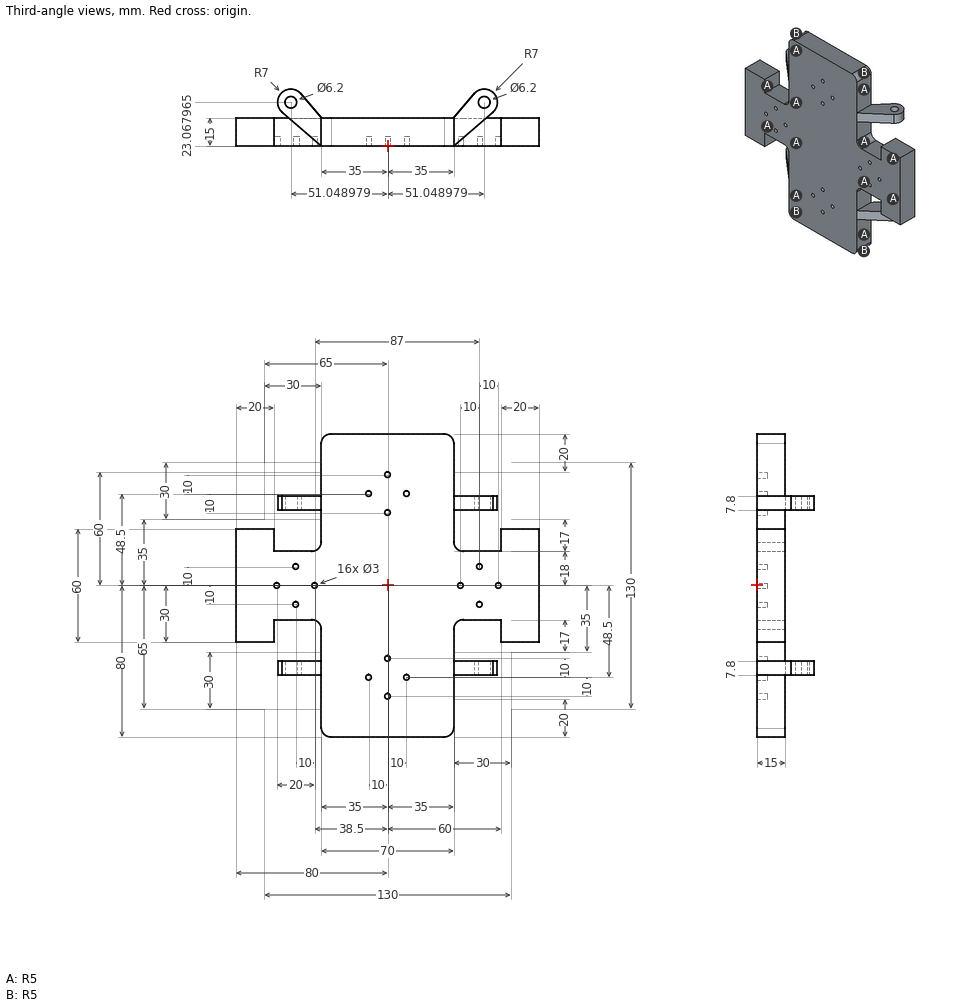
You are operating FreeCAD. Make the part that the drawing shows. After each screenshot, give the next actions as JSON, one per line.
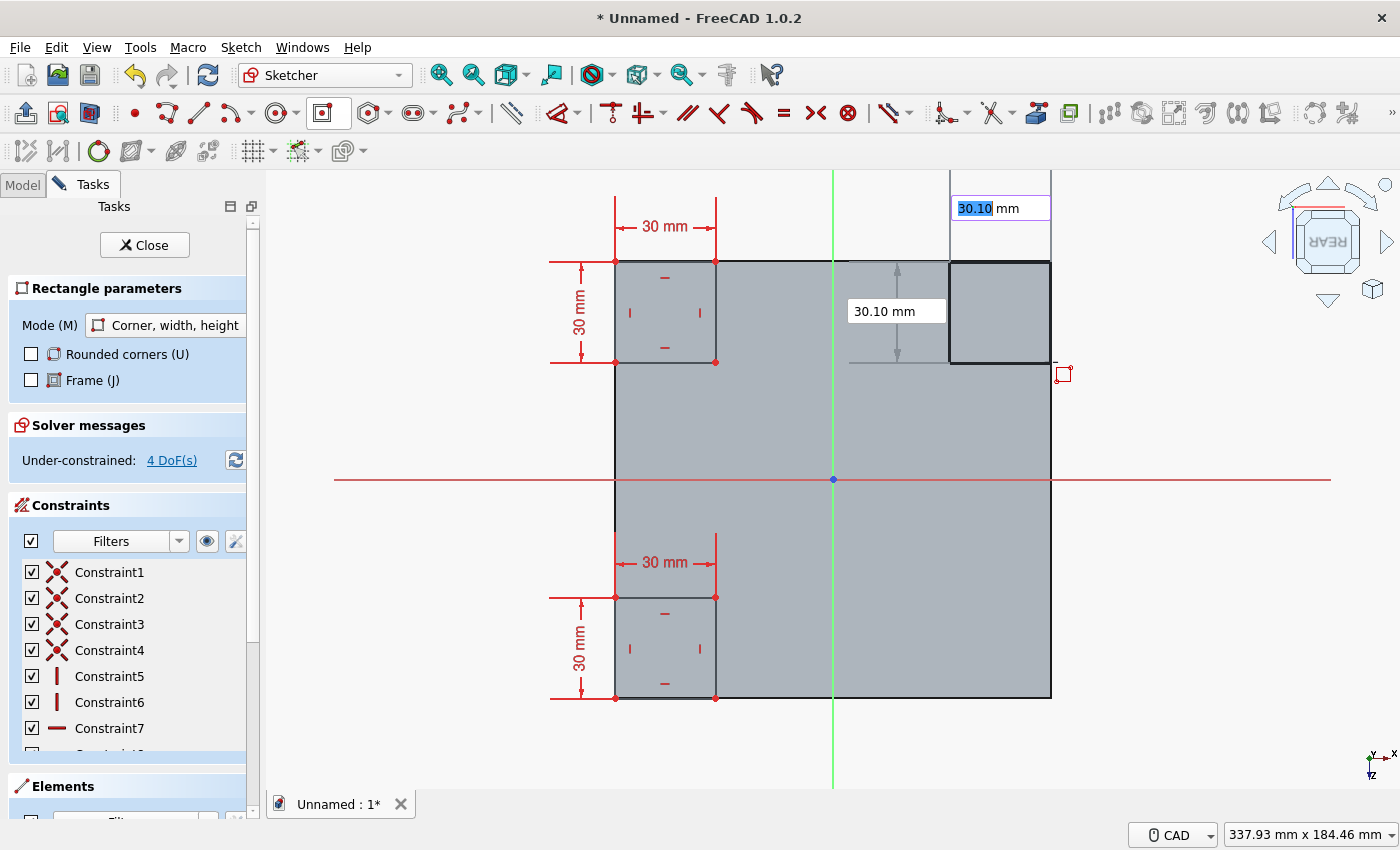
{"action": "type", "text": "30"}
{"action": "key", "text": "Tab"}
{"action": "type", "text": "30"}
{"action": "key", "text": "Return"}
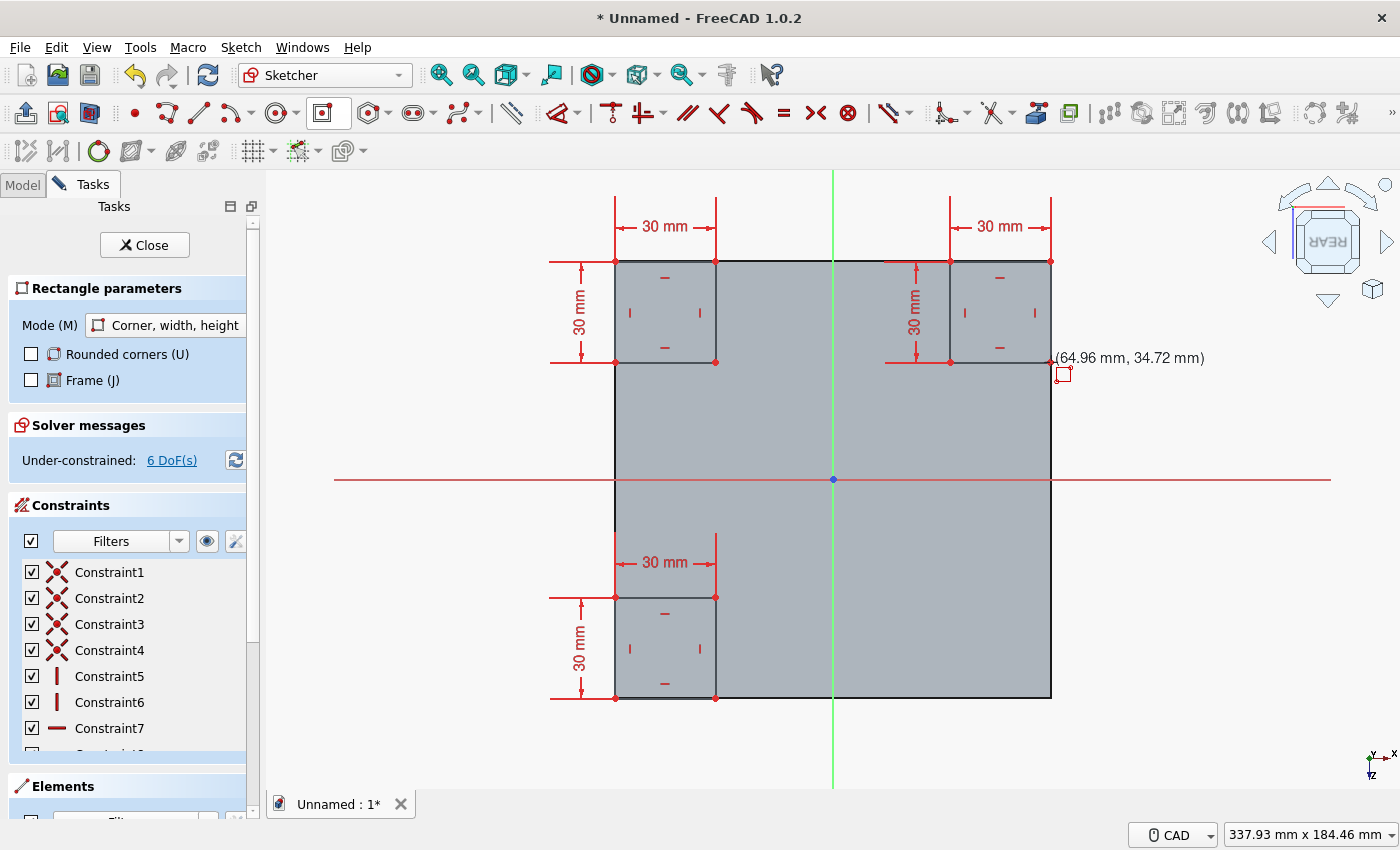
{"action": "left_click", "coordinate": [950, 597]}
{"action": "mouse_move", "coordinate": [1051, 698]}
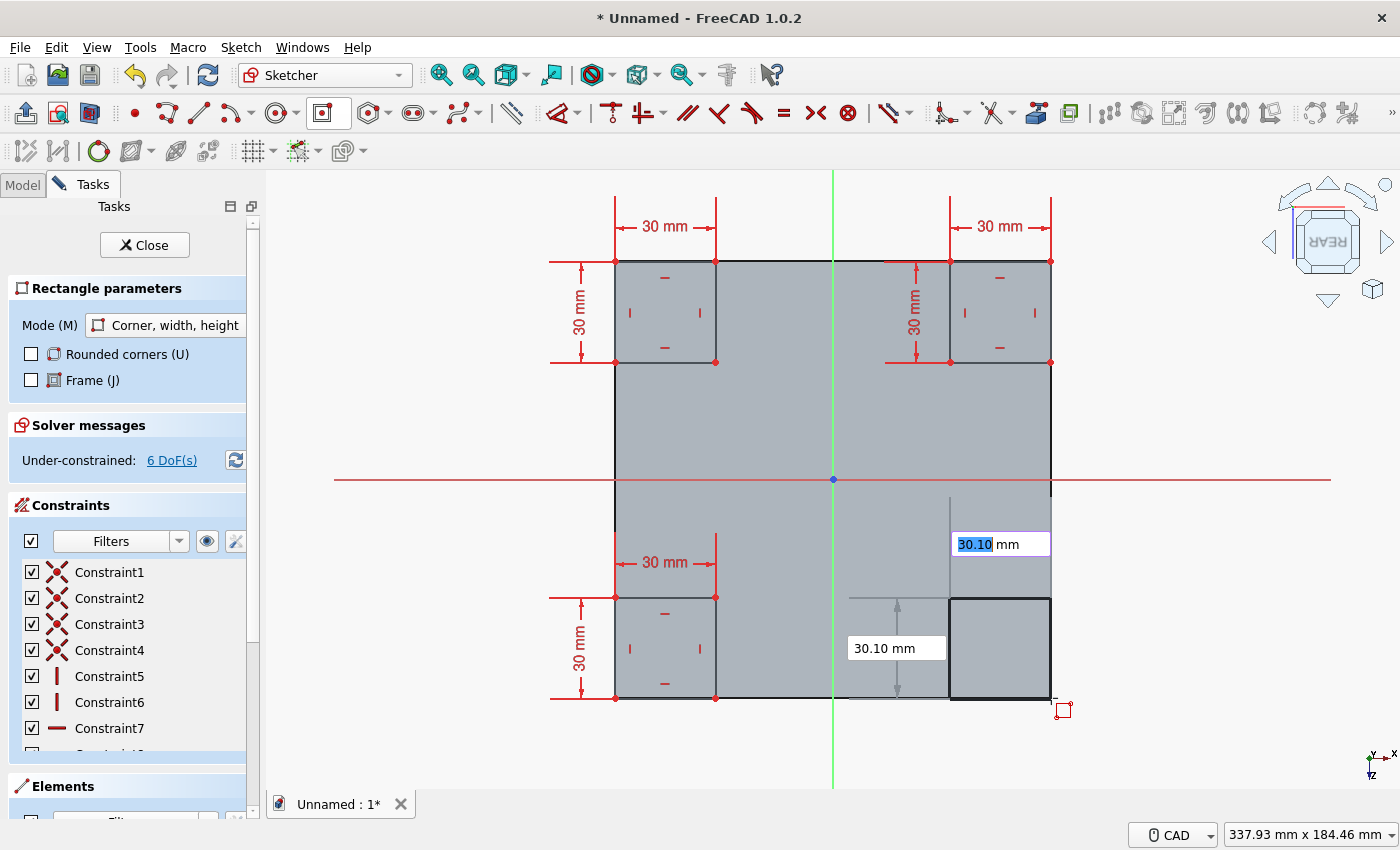
{"action": "type", "text": "30"}
{"action": "key", "text": "Tab"}
{"action": "type", "text": "30"}
{"action": "key", "text": "Return"}
{"action": "key", "text": "Escape"}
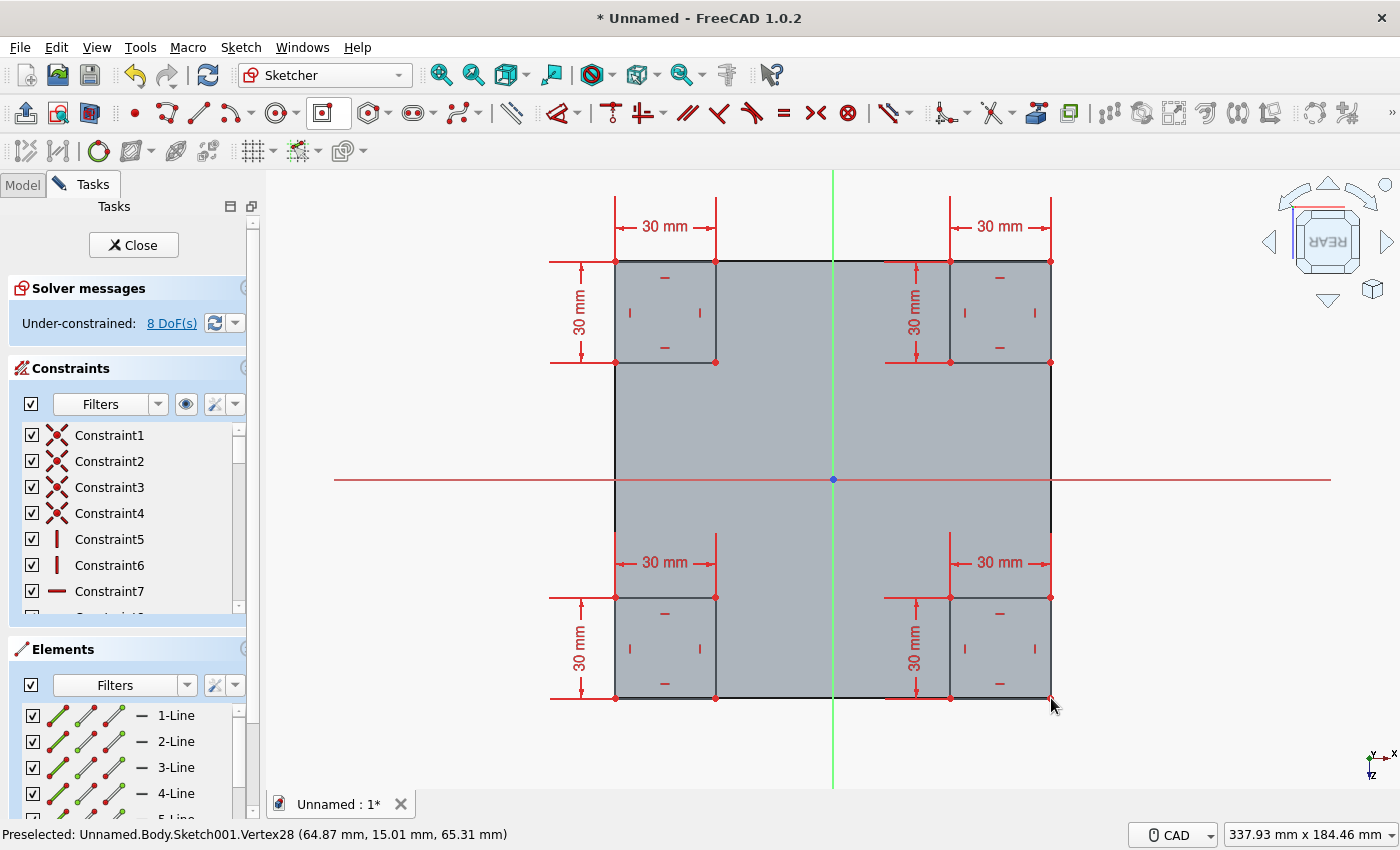
{"action": "key", "text": "d"}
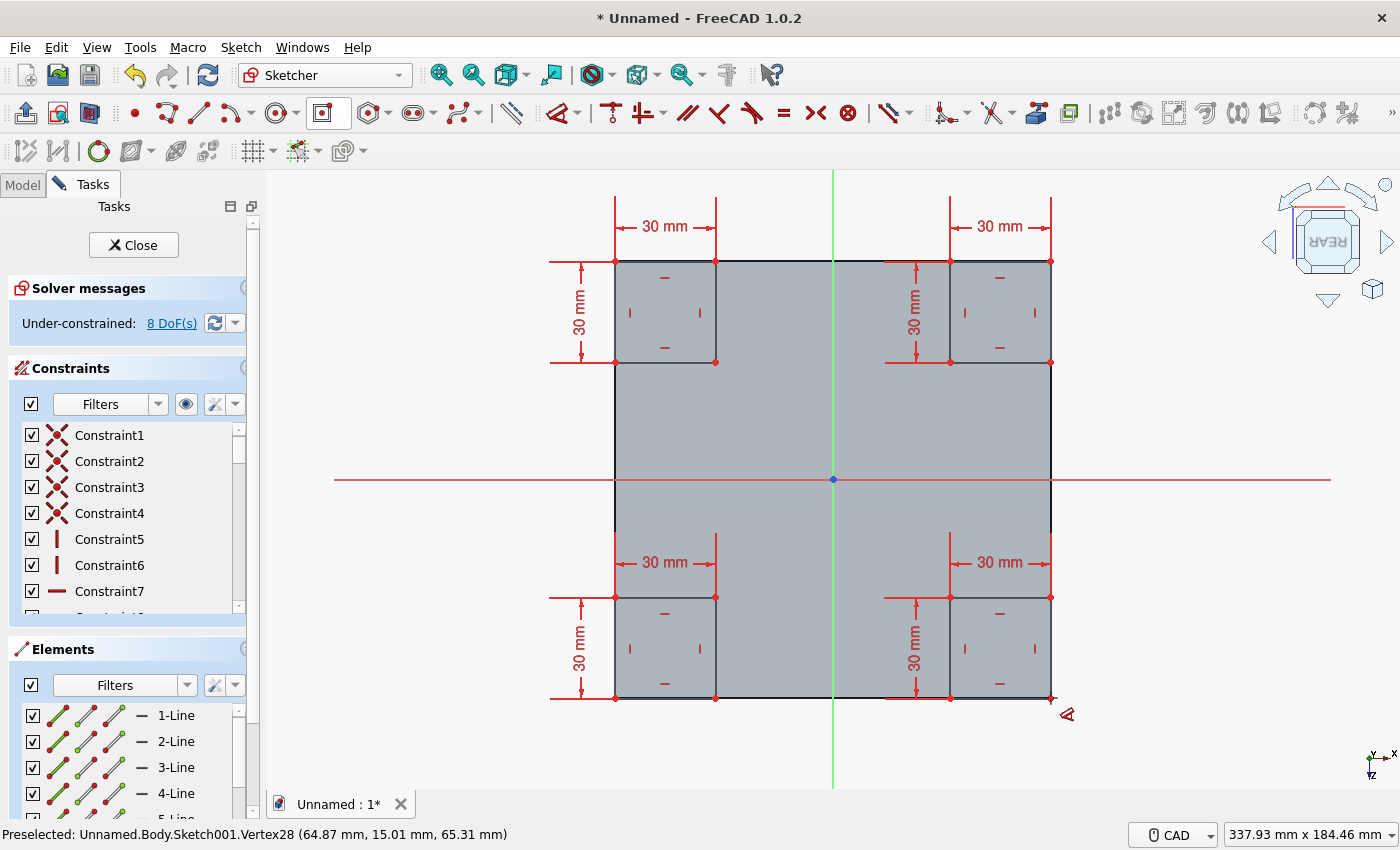
{"action": "left_click", "coordinate": [615, 598]}
{"action": "left_click", "coordinate": [674, 632]}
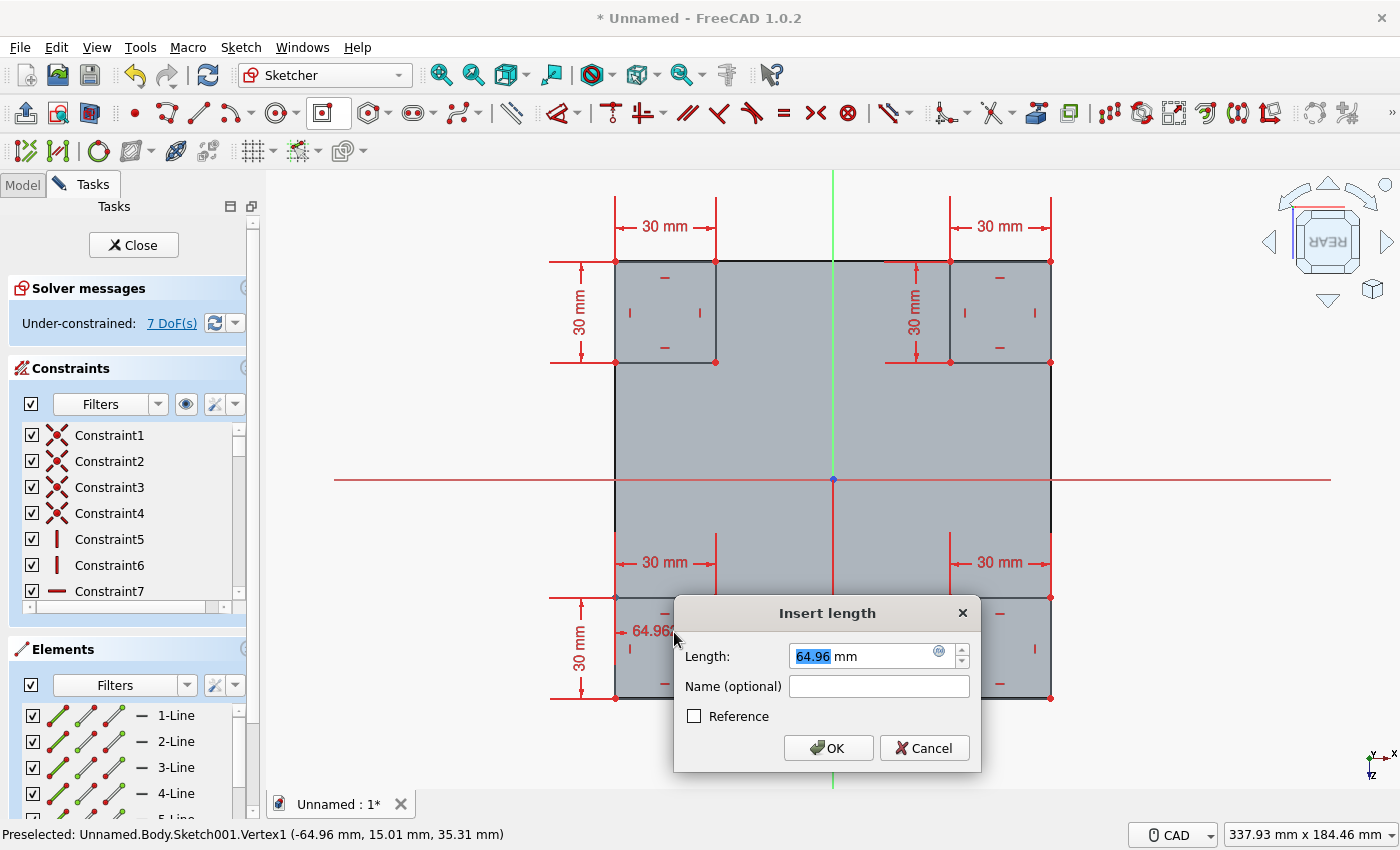
{"action": "type", "text": "65"}
{"action": "key", "text": "Return"}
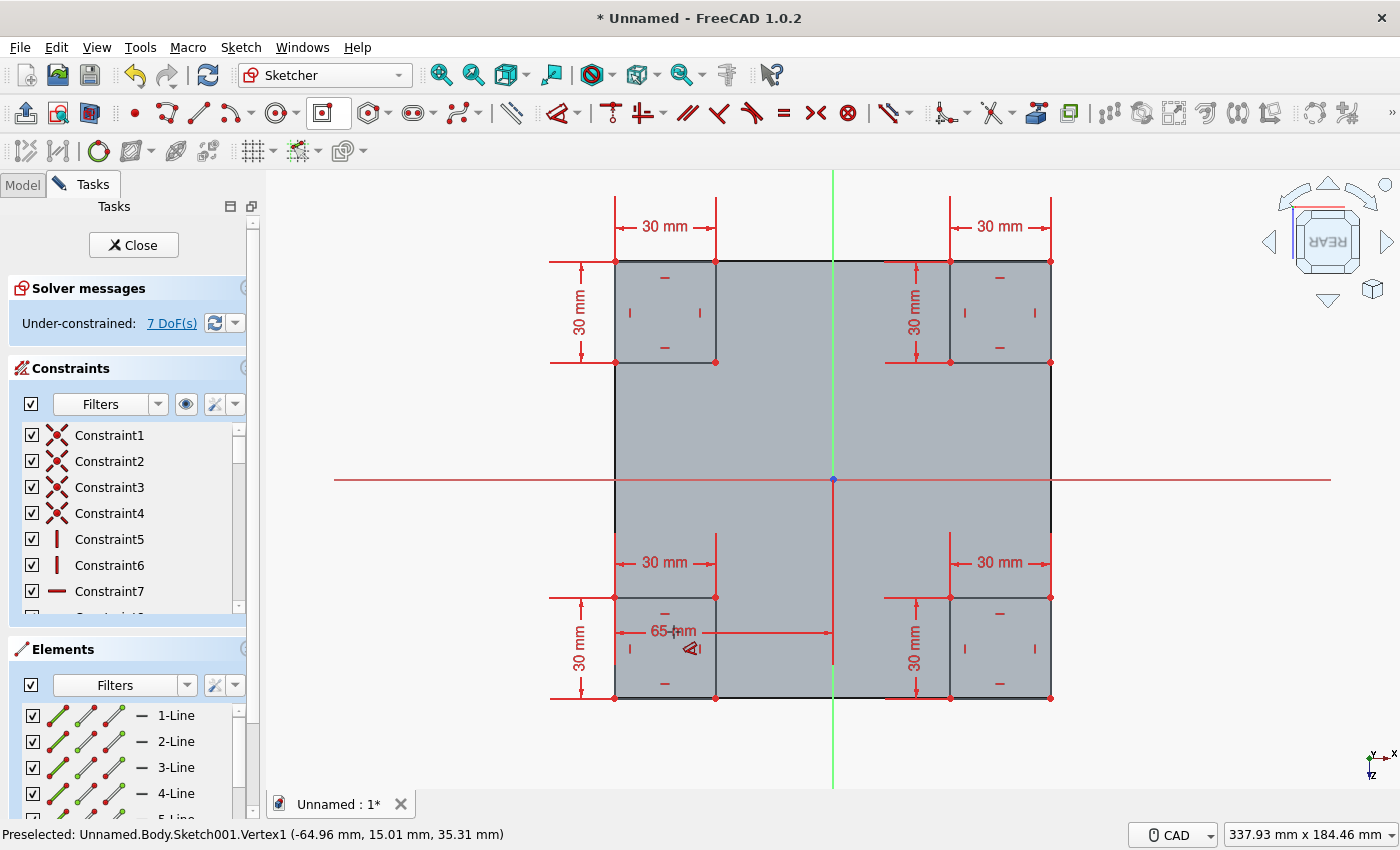
{"action": "left_click", "coordinate": [615, 598]}
{"action": "left_click", "coordinate": [581, 539]}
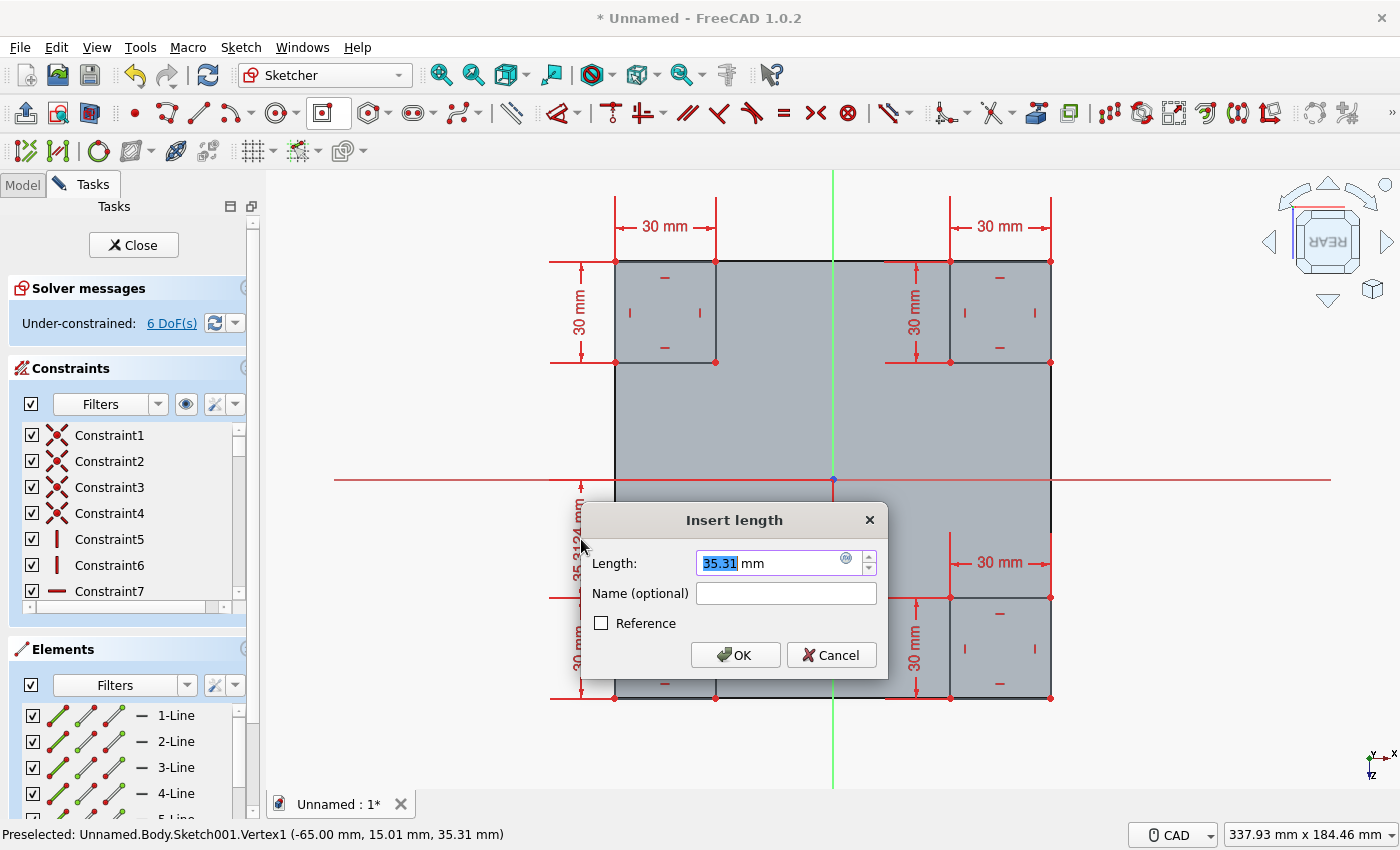
{"action": "type", "text": "35"}
{"action": "key", "text": "Return"}